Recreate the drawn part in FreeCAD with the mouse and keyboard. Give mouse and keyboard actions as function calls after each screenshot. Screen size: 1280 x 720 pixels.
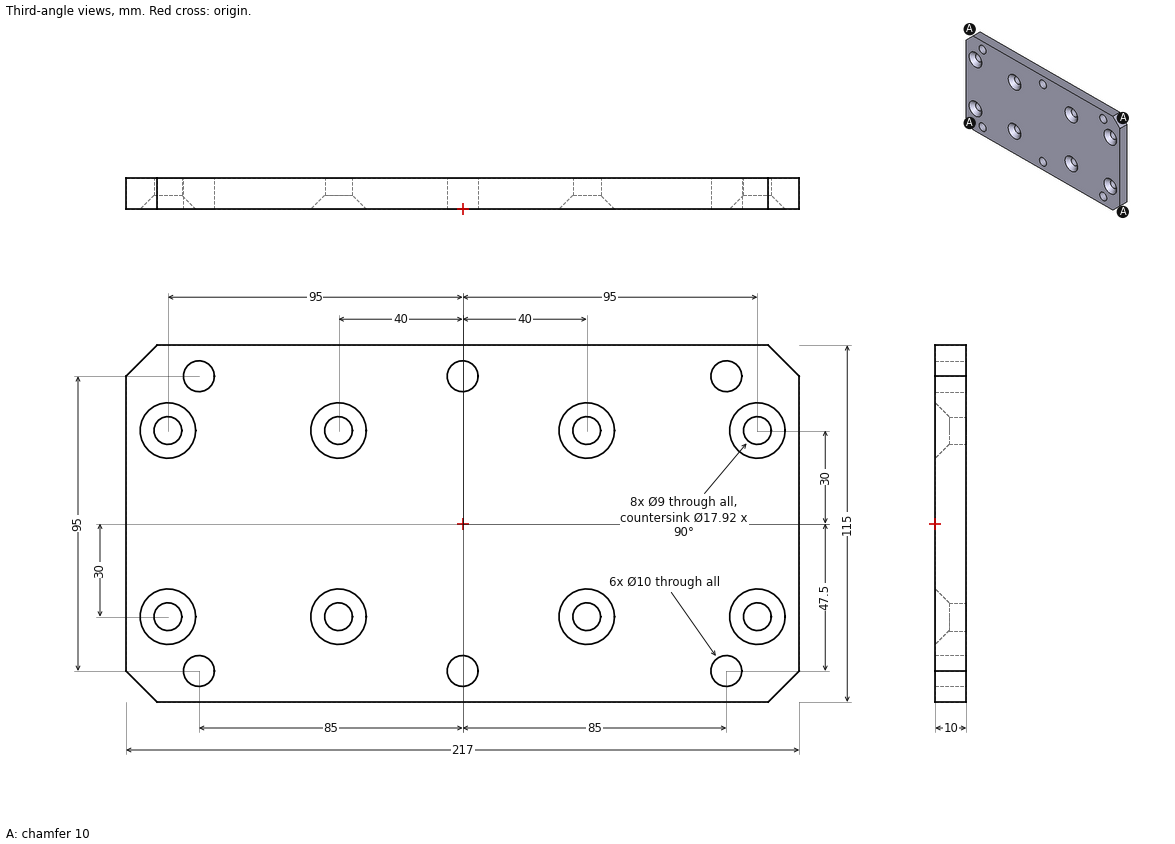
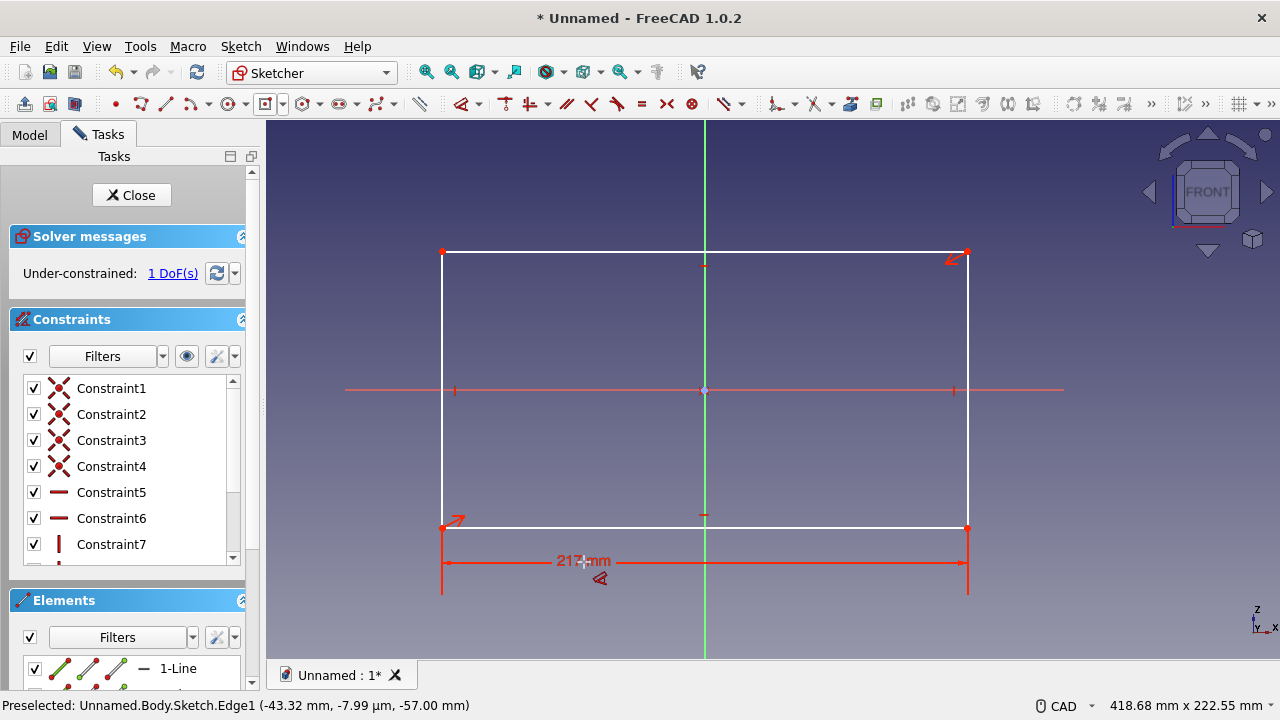
click(968, 445)
click(1002, 327)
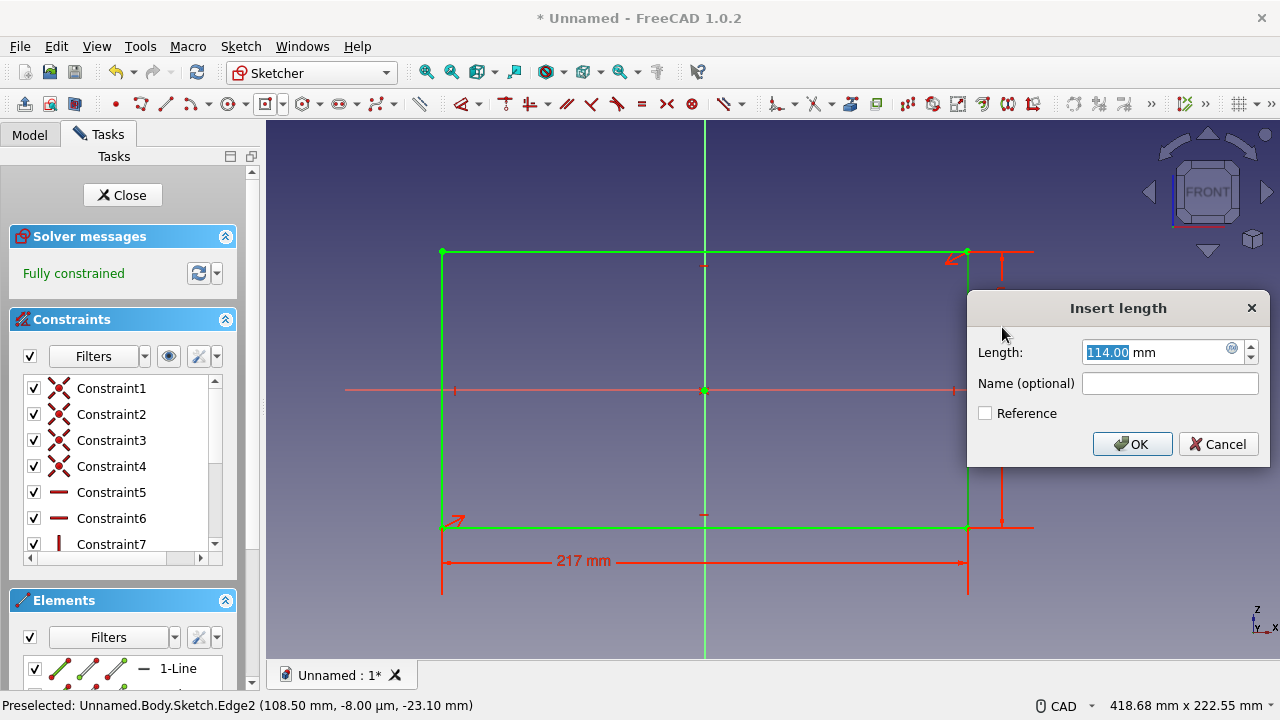
text(115)
key(Return)
key(Escape)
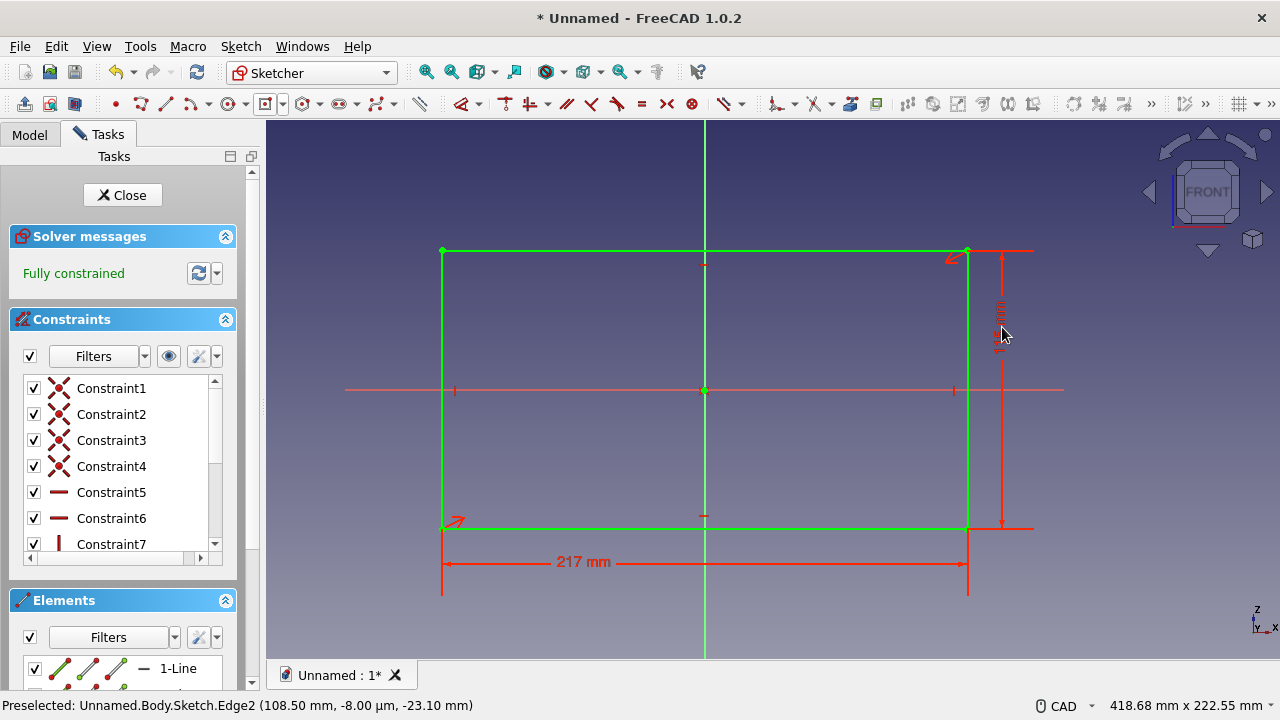
click(123, 195)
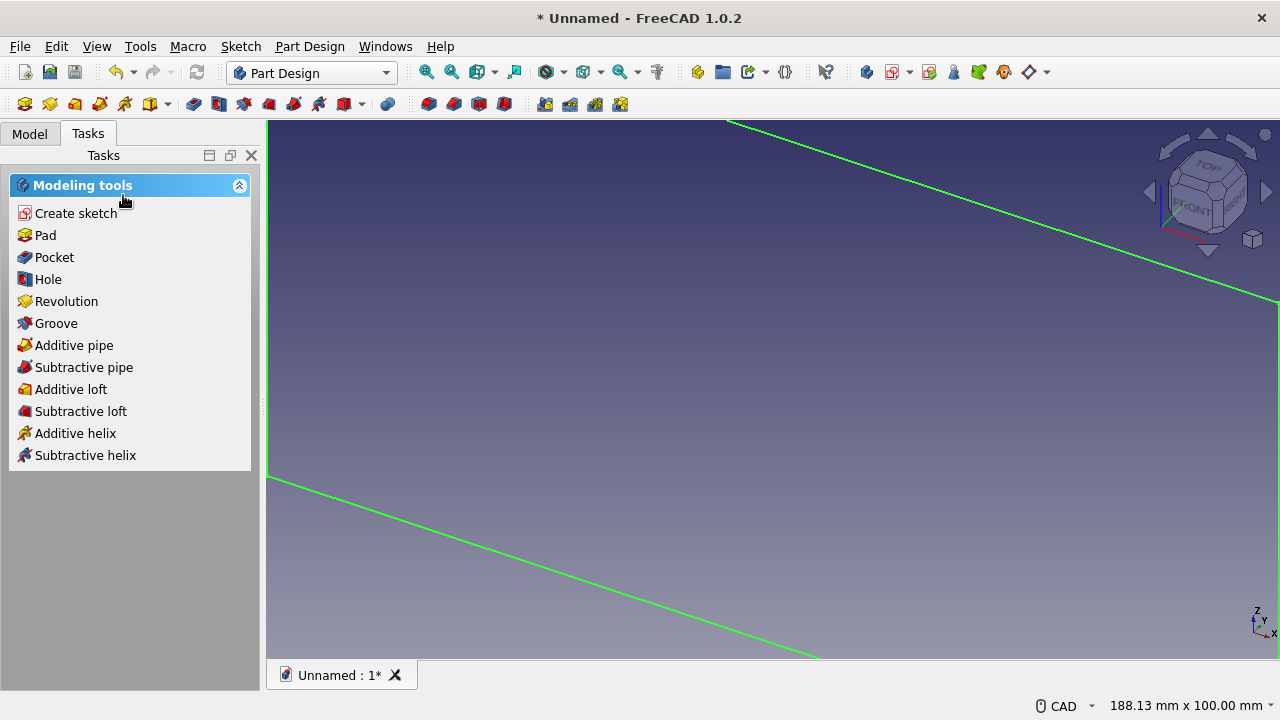
click(25, 104)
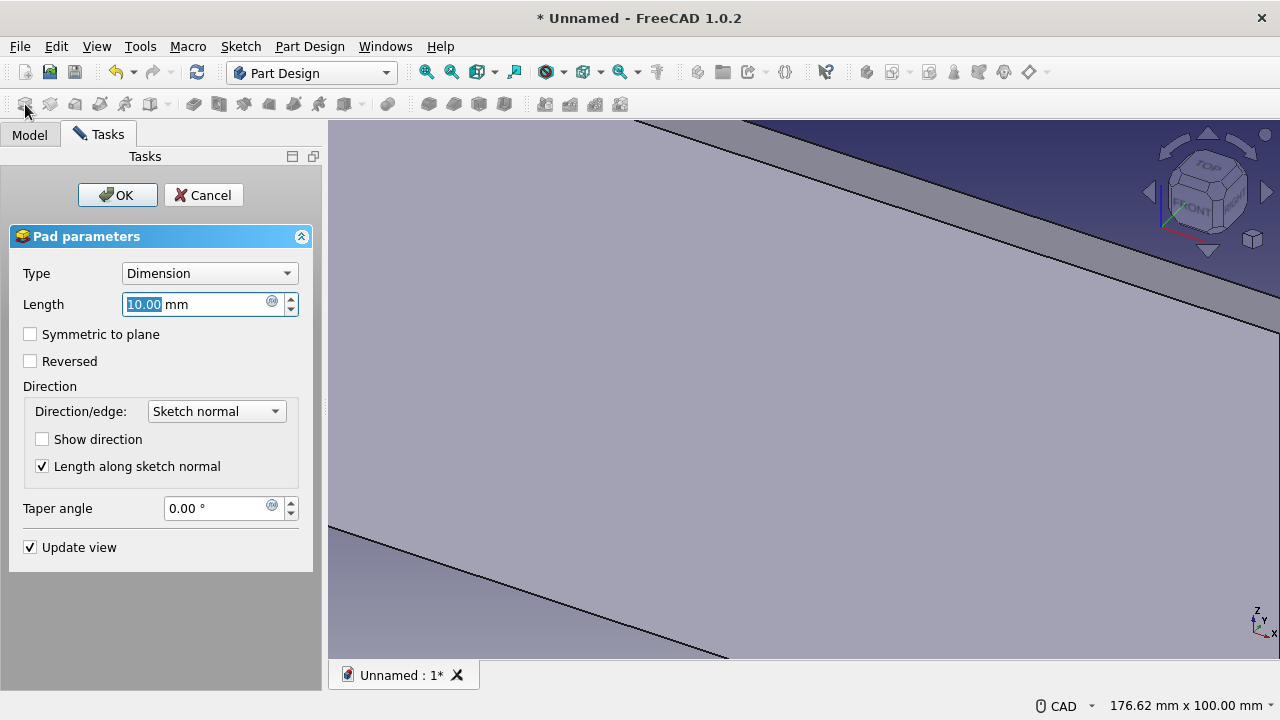
text(10)
key(Tab)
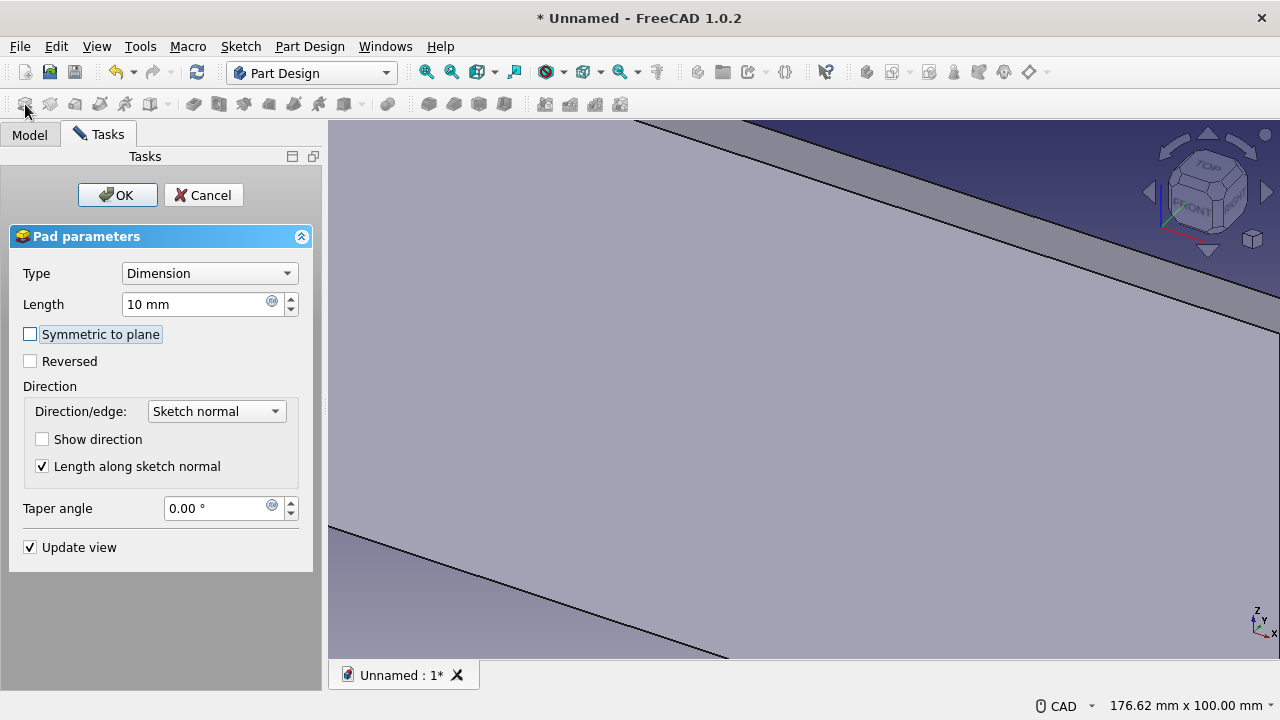
click(31, 361)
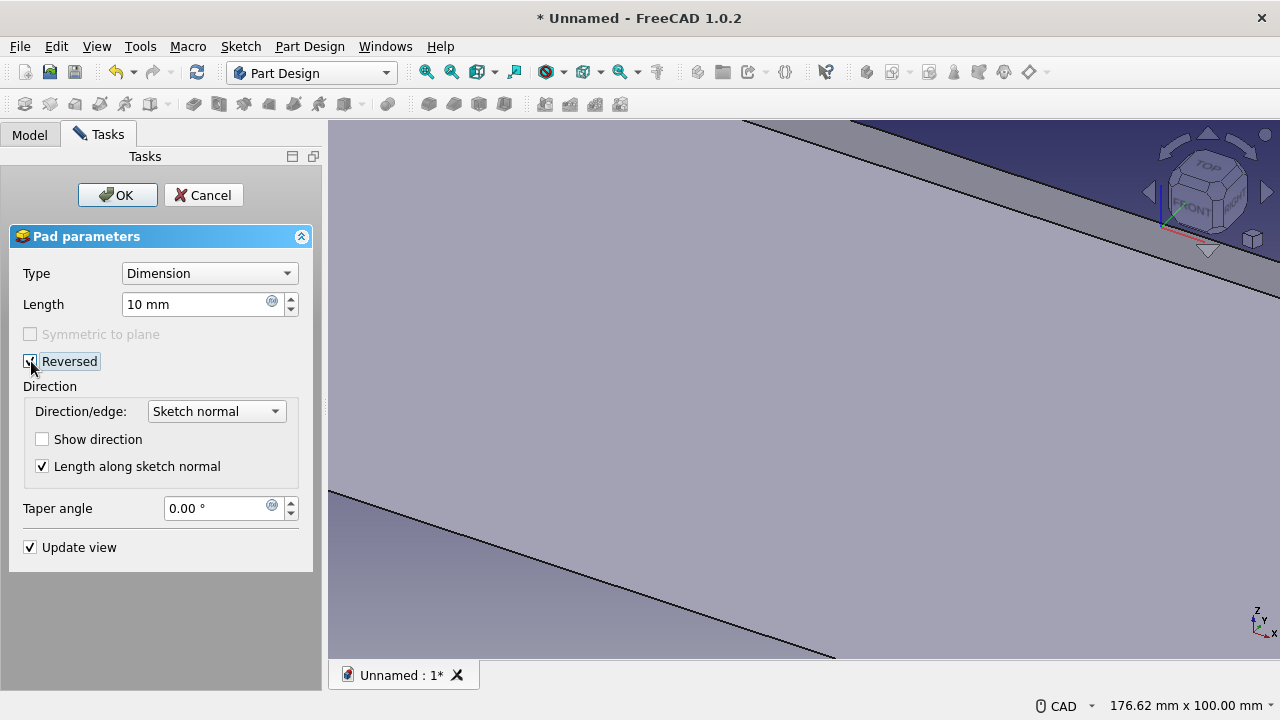
click(118, 195)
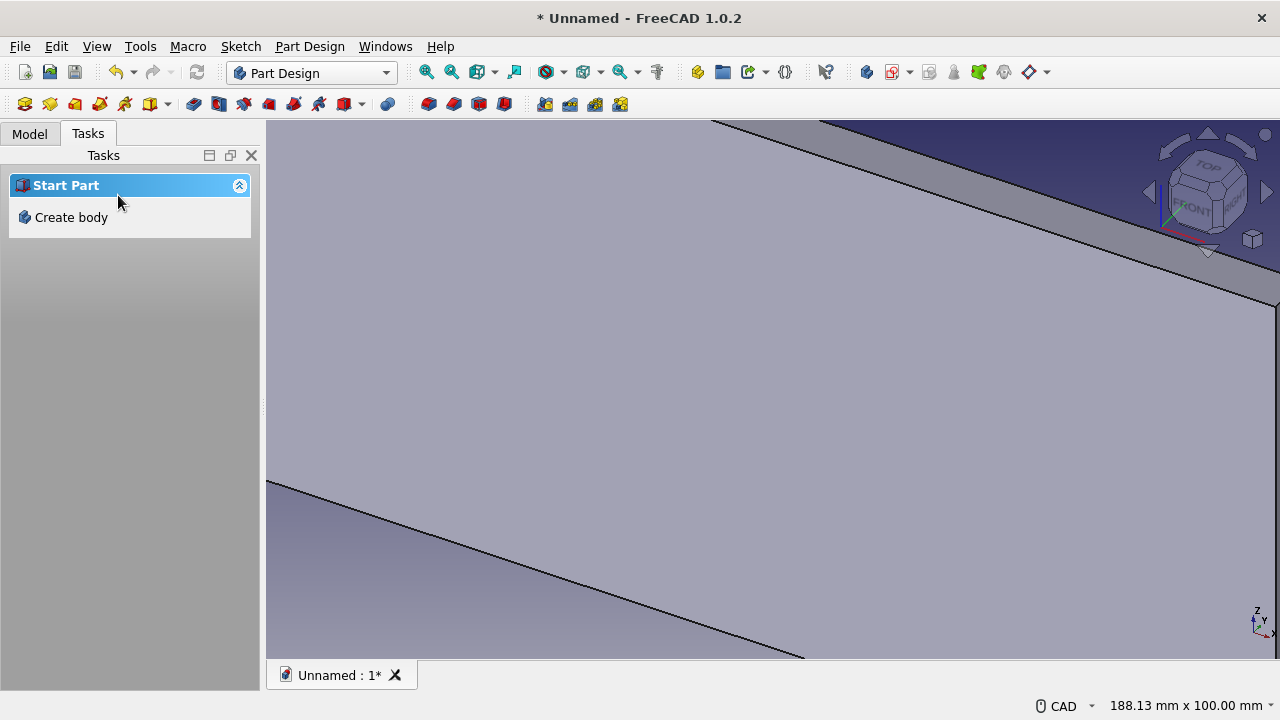
click(427, 72)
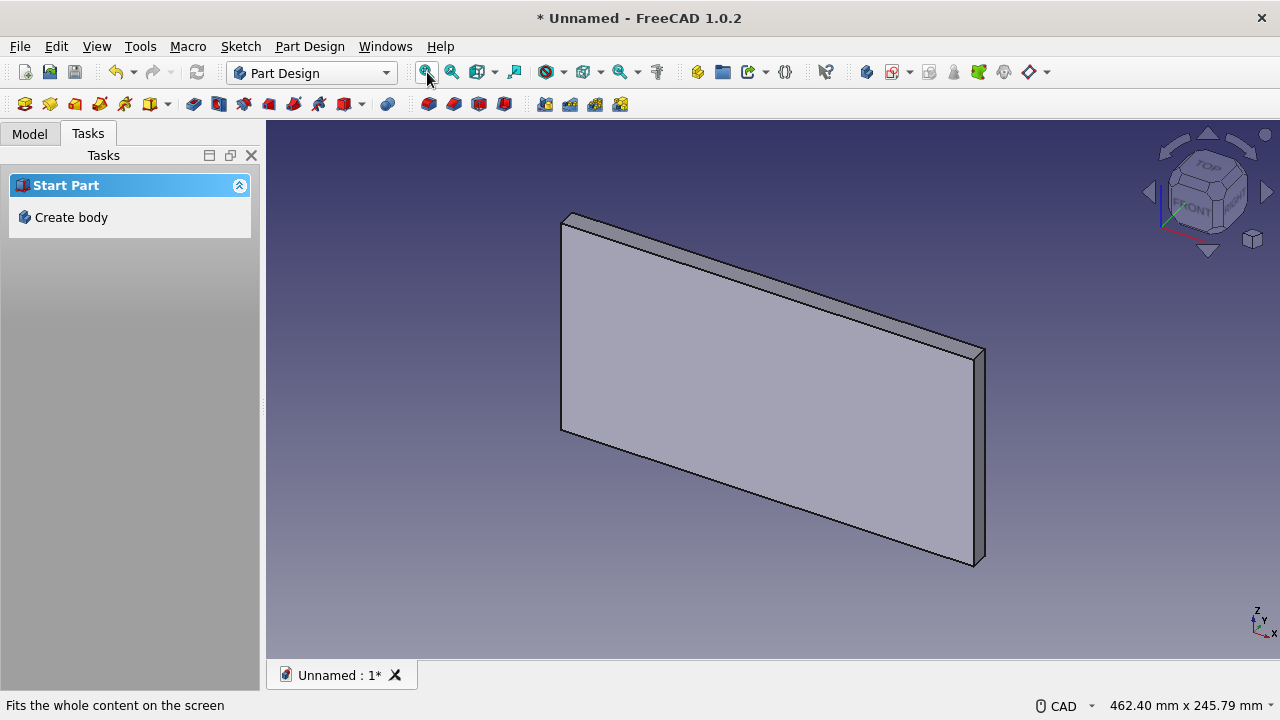
click(826, 413)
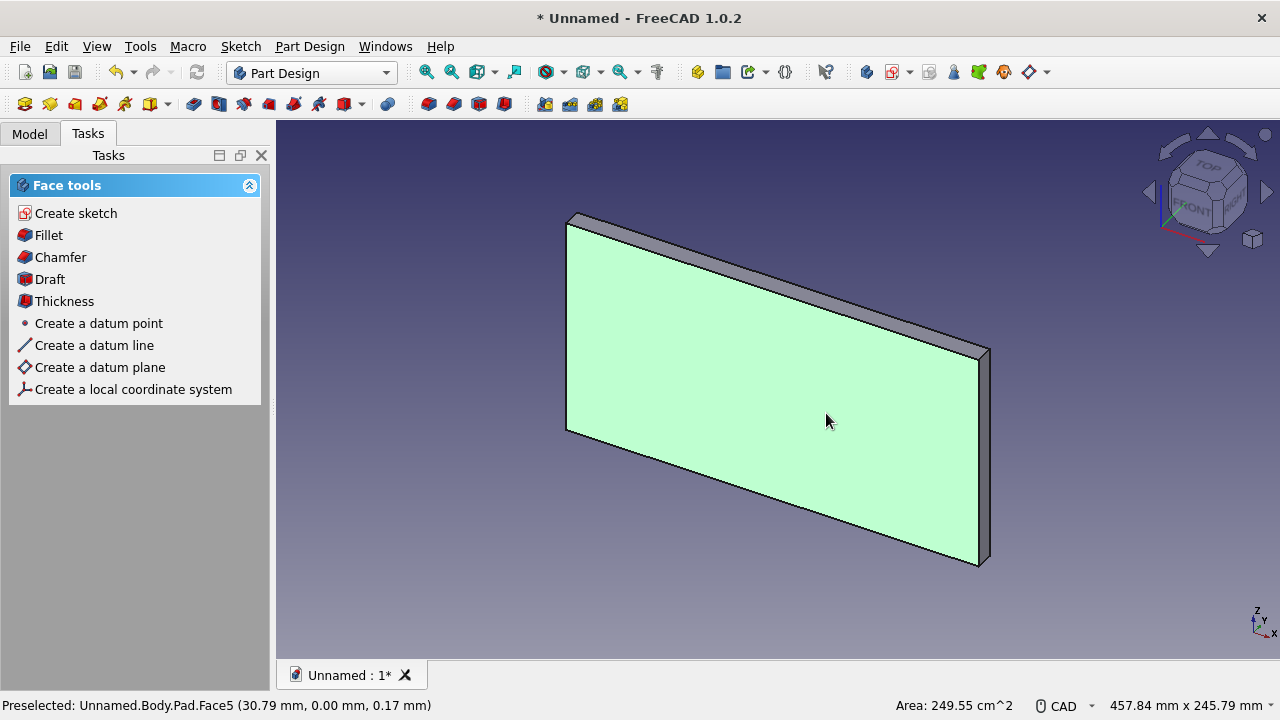
click(892, 72)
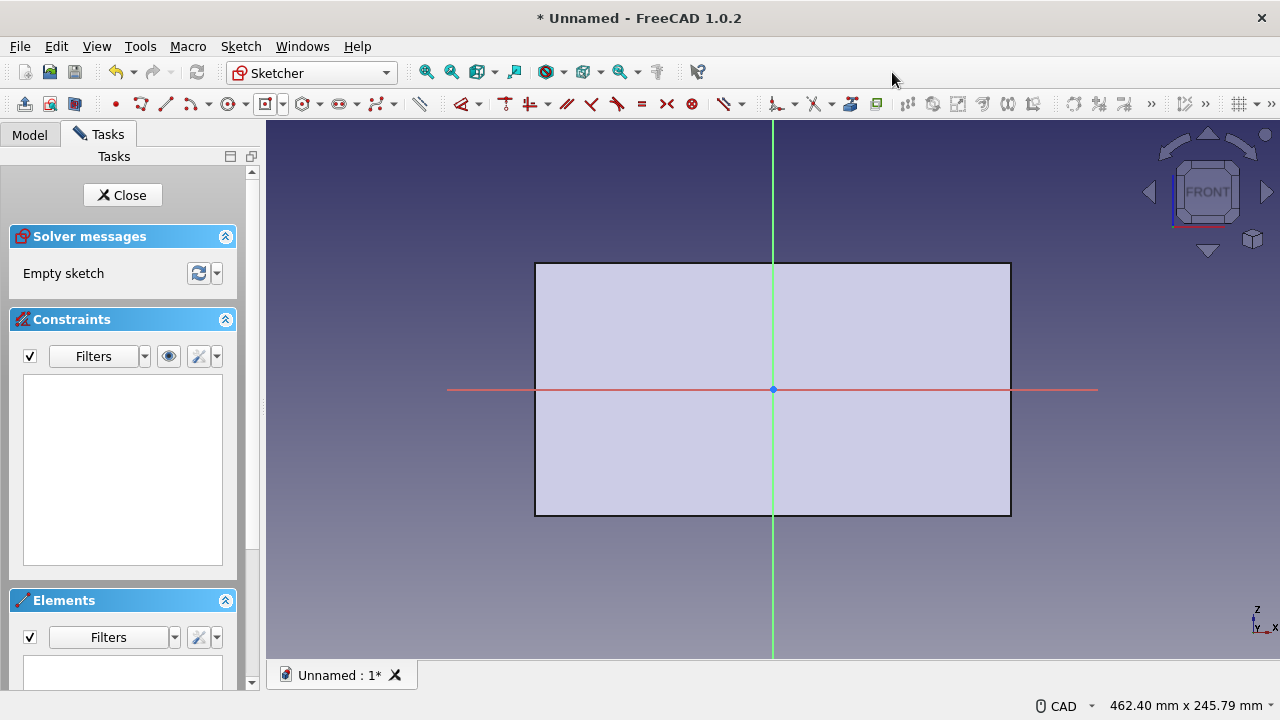
click(228, 104)